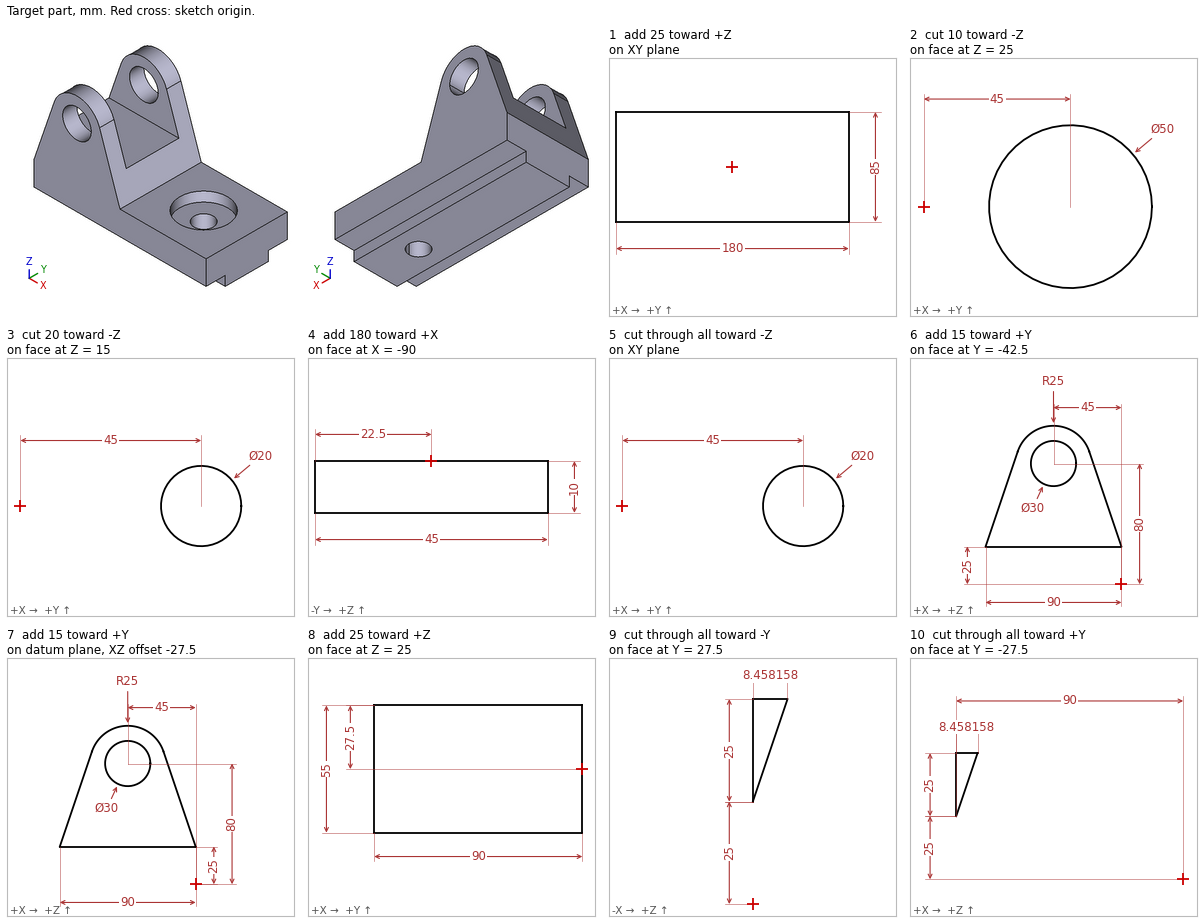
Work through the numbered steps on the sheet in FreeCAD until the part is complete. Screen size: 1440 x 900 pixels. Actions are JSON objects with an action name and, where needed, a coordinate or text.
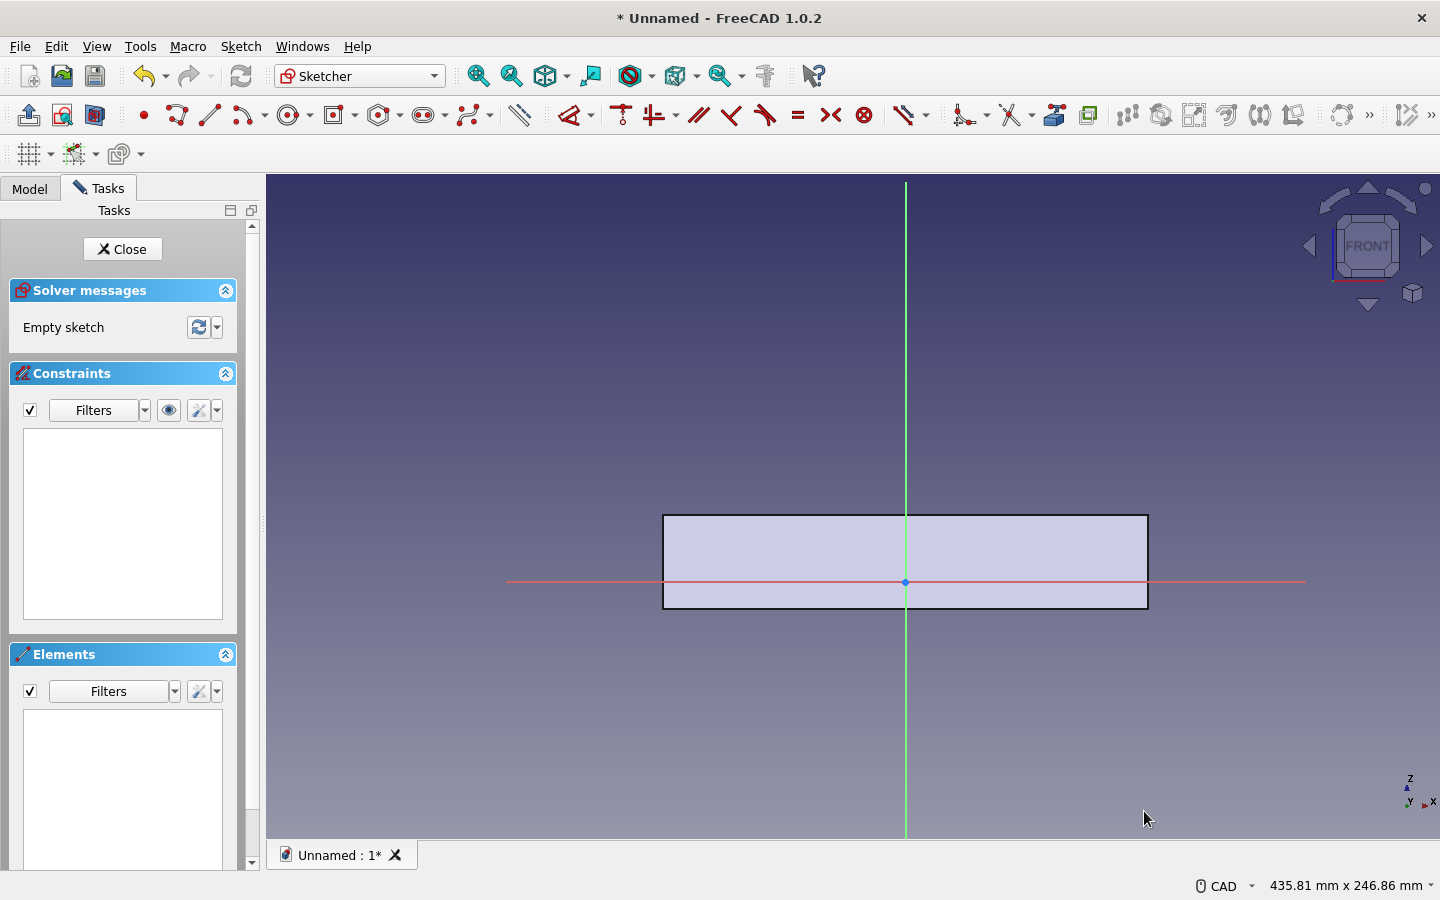
{"action": "scroll", "coordinate": [785, 307], "scroll_direction": "up", "scroll_amount": 2}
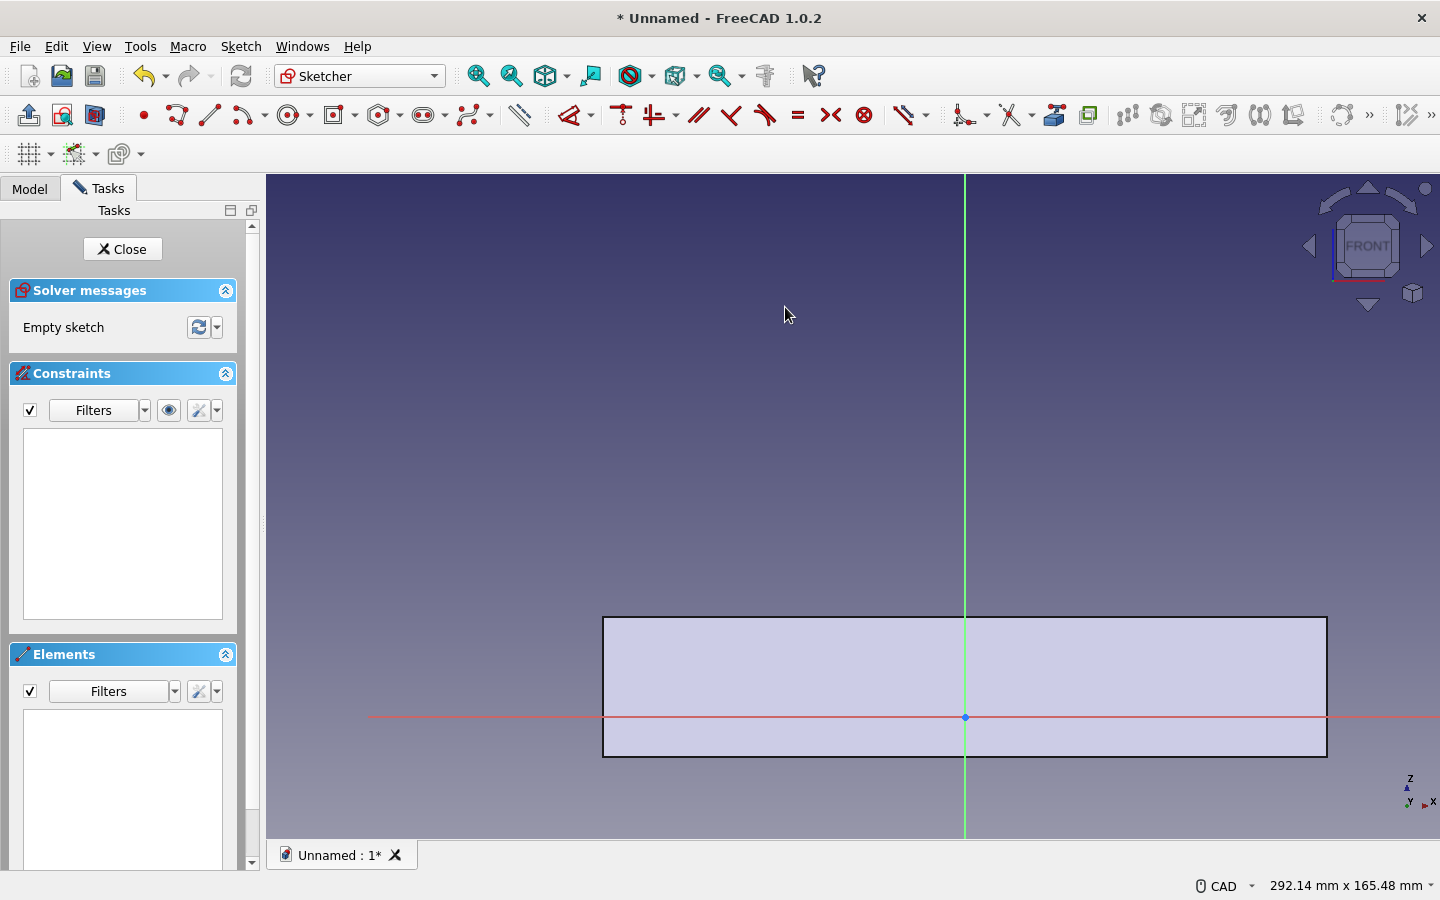
{"action": "left_click", "coordinate": [177, 116]}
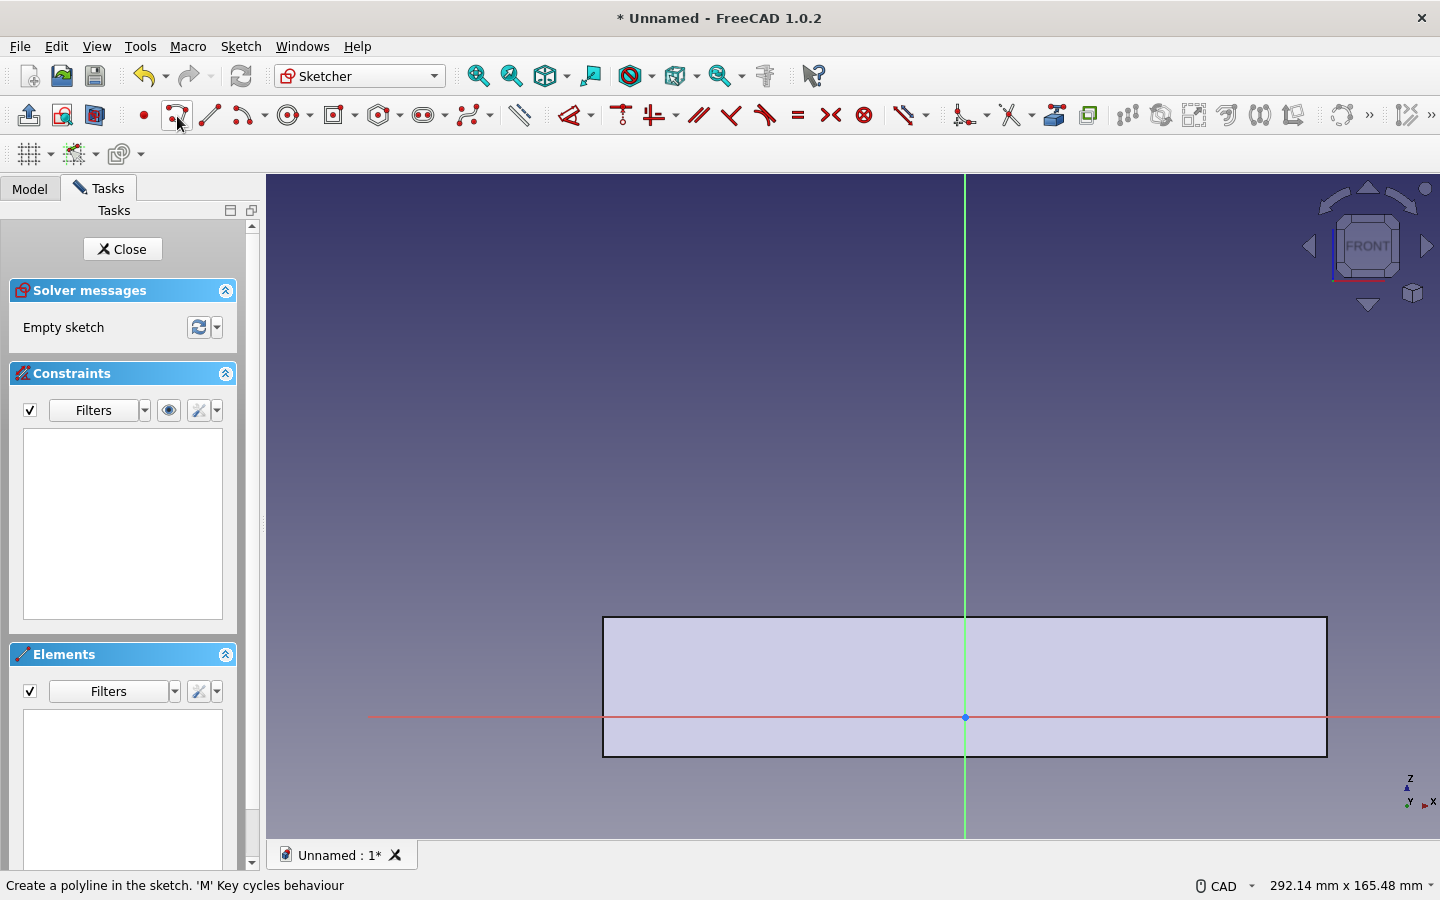
{"action": "left_click", "coordinate": [689, 364]}
{"action": "left_click", "coordinate": [603, 617]}
{"action": "left_click", "coordinate": [965, 617]}
{"action": "left_click", "coordinate": [879, 364]}
{"action": "right_click", "coordinate": [879, 364]}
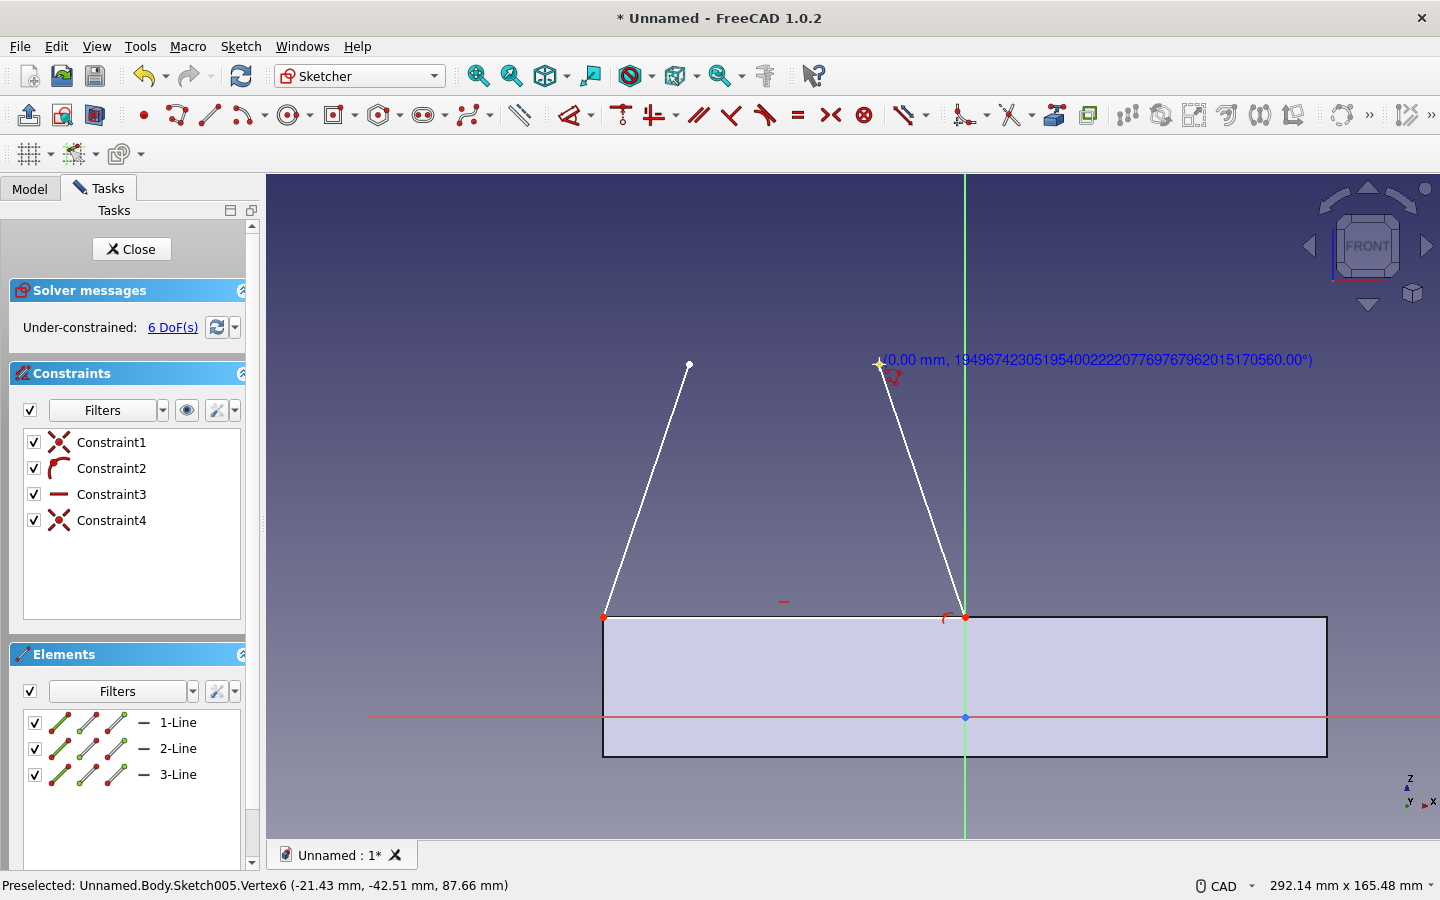
{"action": "left_click", "coordinate": [264, 116]}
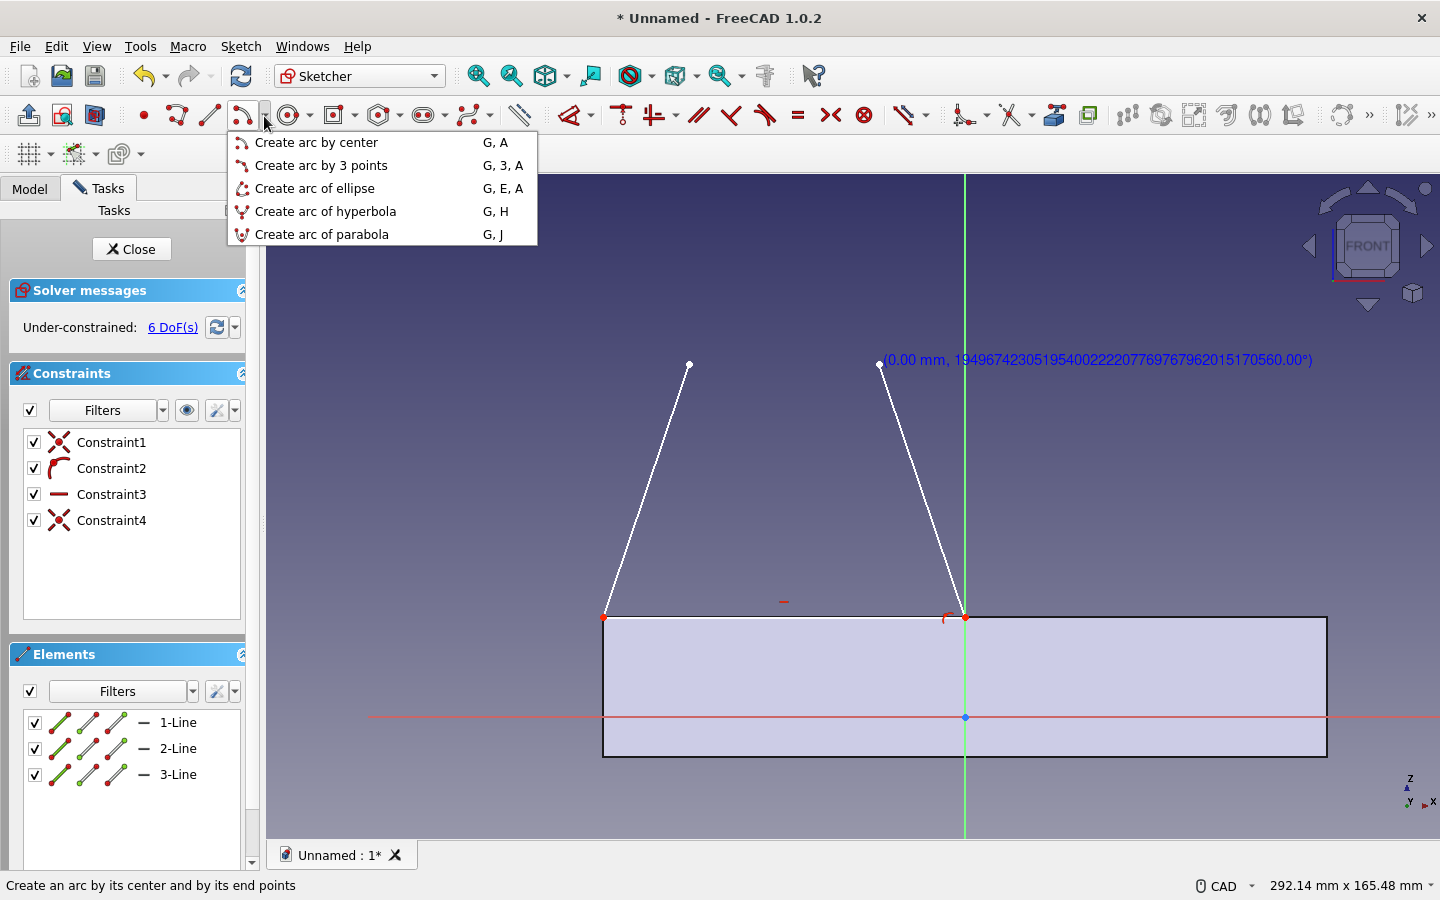
{"action": "left_click", "coordinate": [382, 166]}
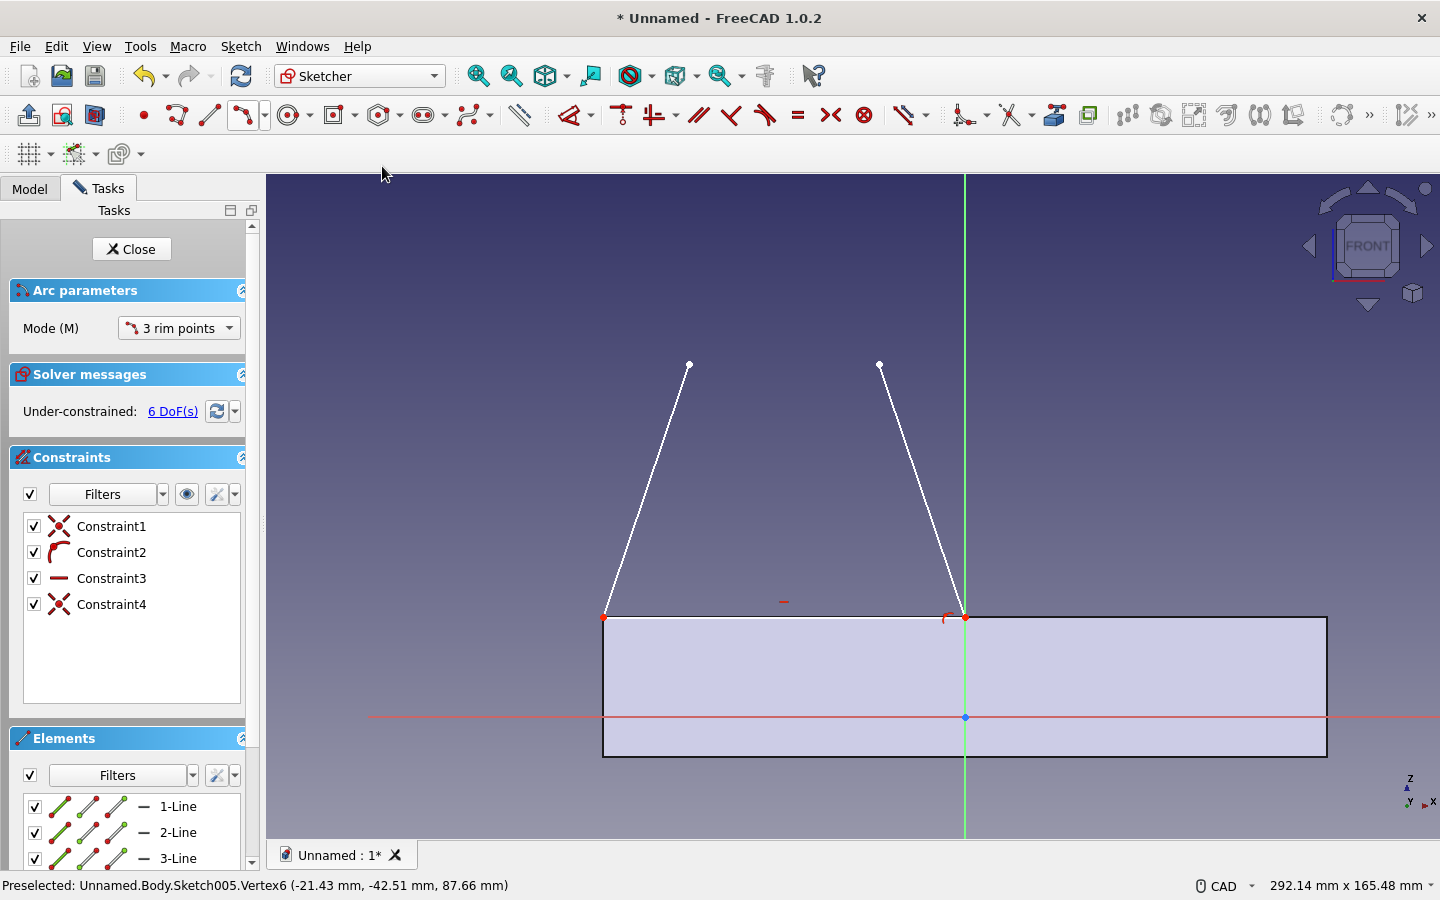
{"action": "left_click", "coordinate": [879, 365]}
{"action": "left_click", "coordinate": [689, 365]}
{"action": "left_click", "coordinate": [784, 295]}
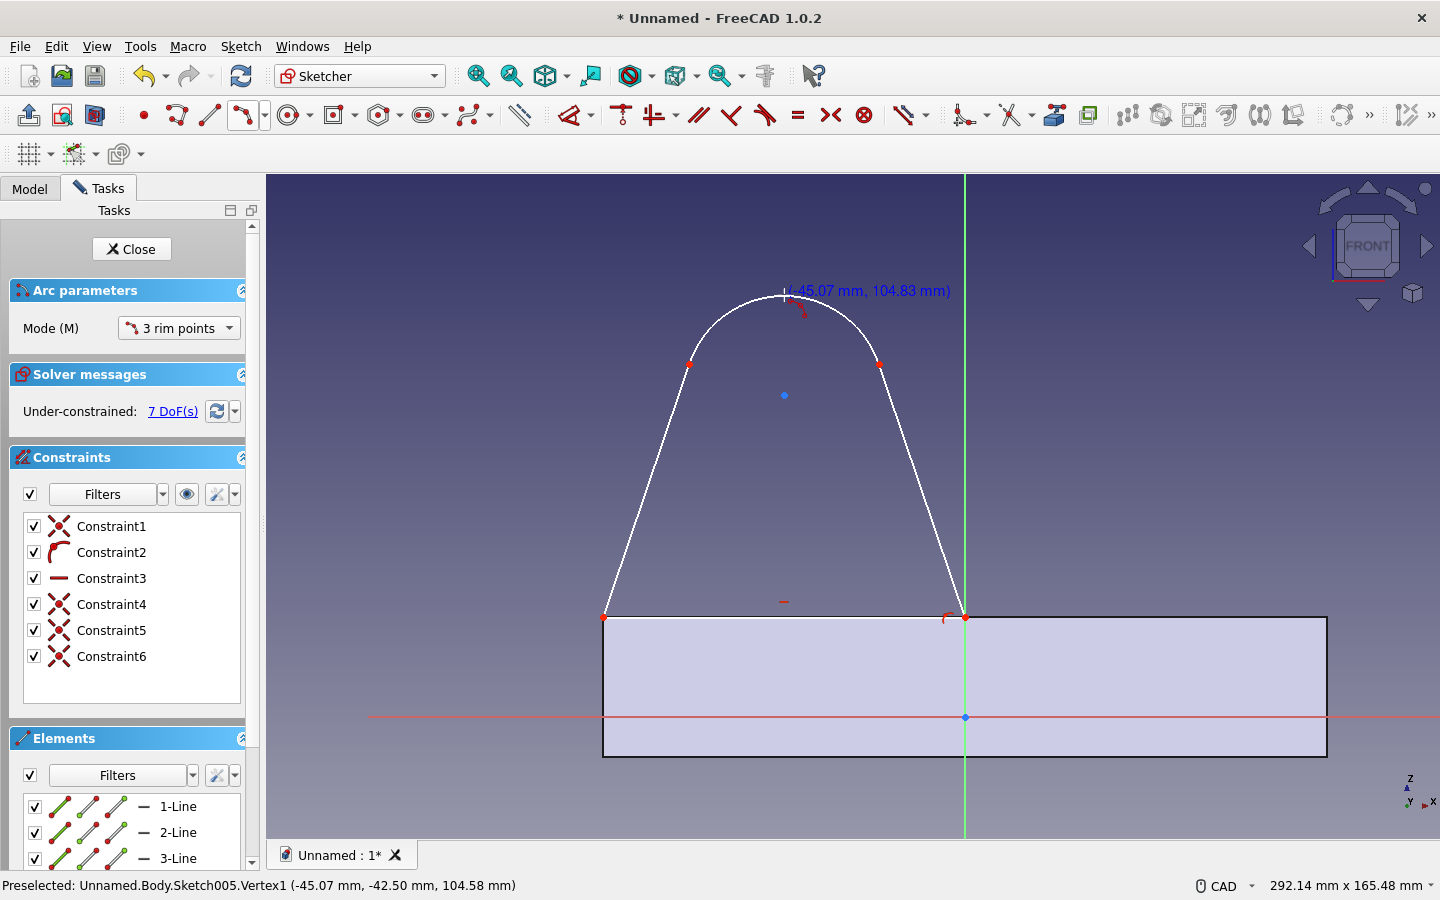
{"action": "left_click", "coordinate": [288, 116]}